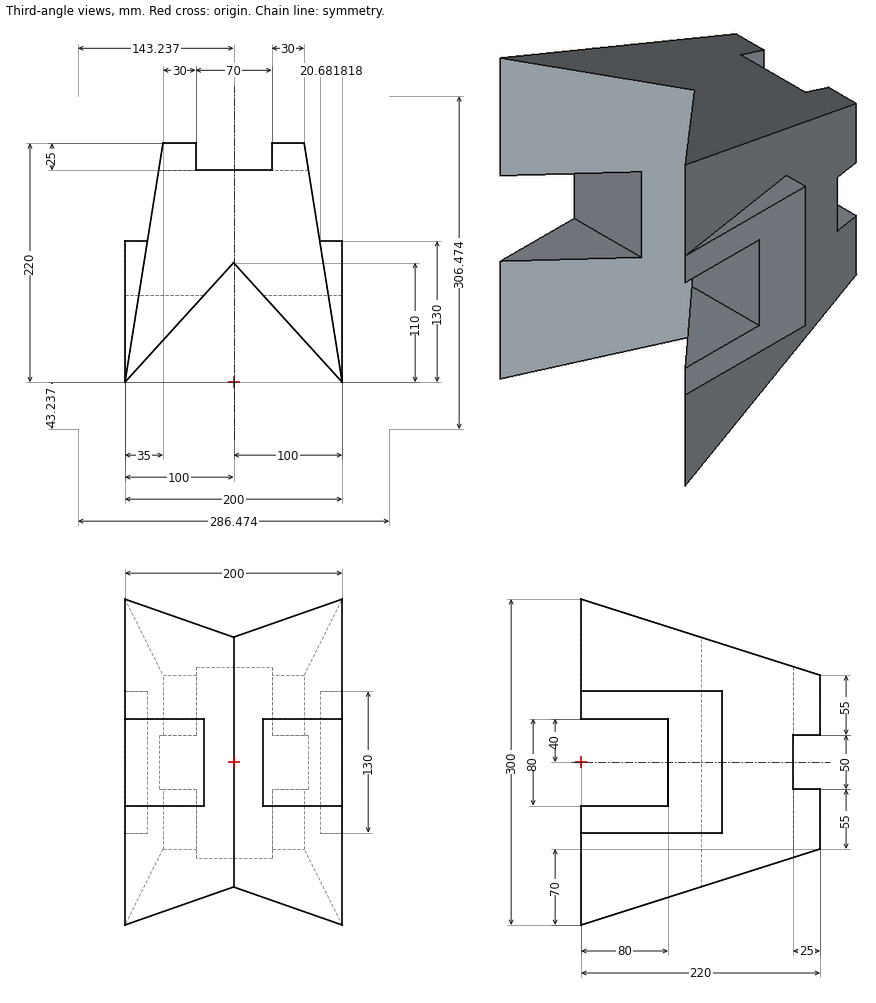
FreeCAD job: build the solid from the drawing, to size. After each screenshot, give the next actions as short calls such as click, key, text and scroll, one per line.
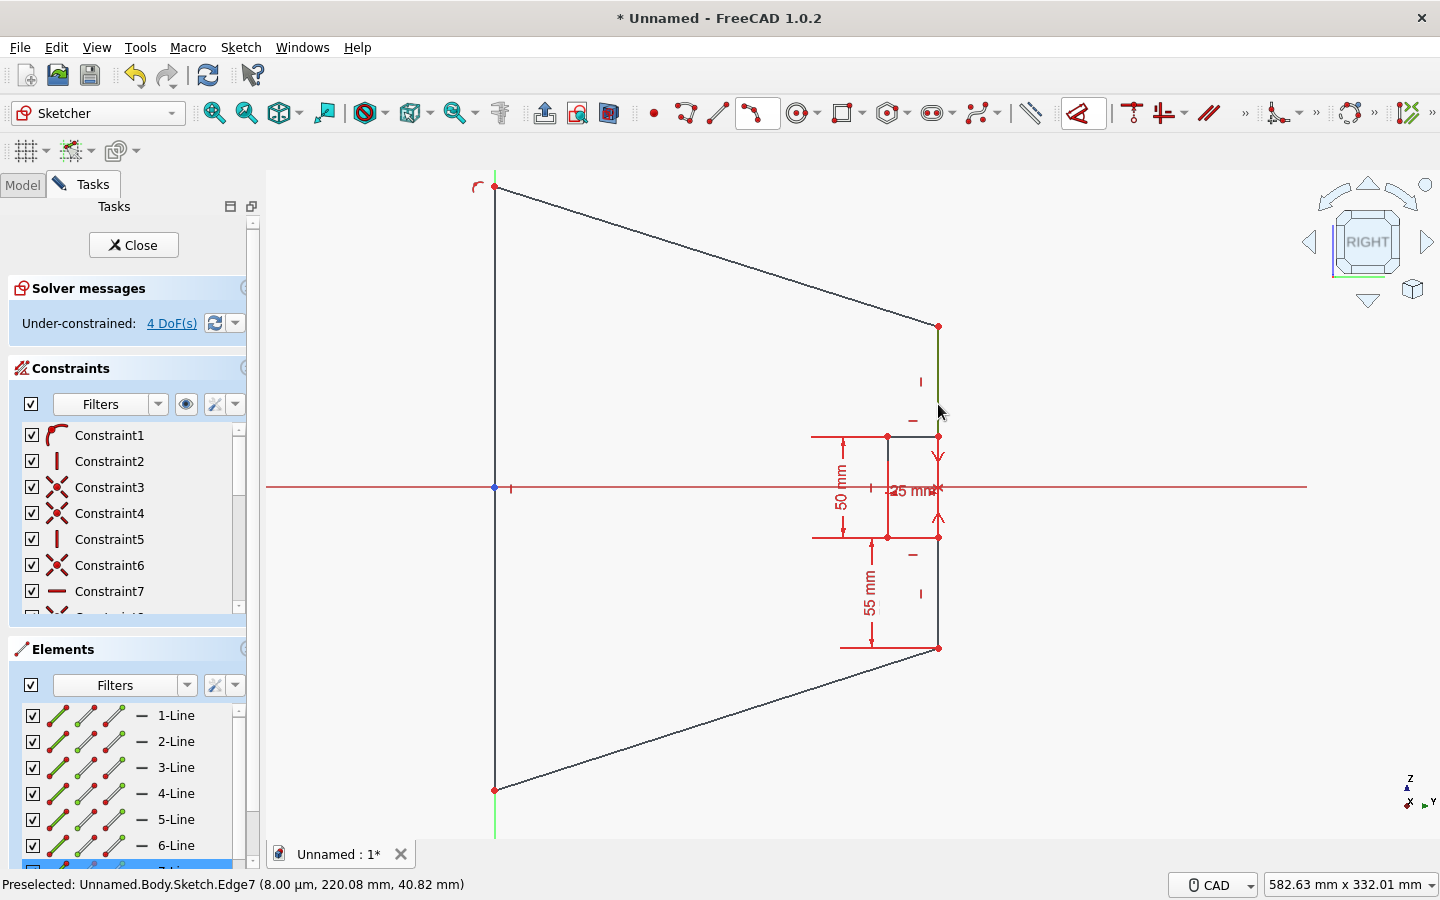
key(i)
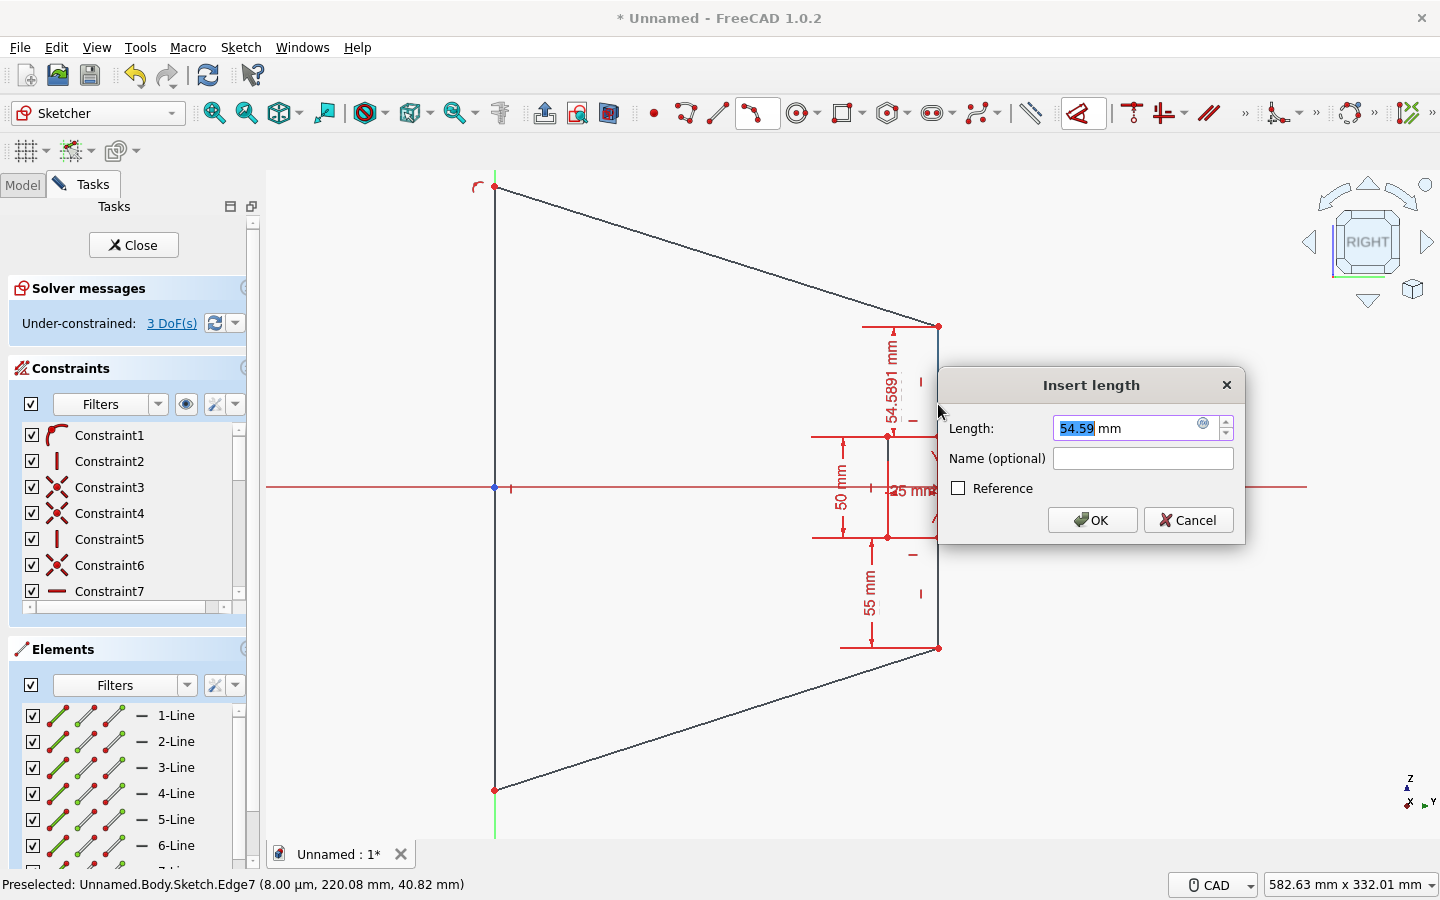
text(55)
key(Return)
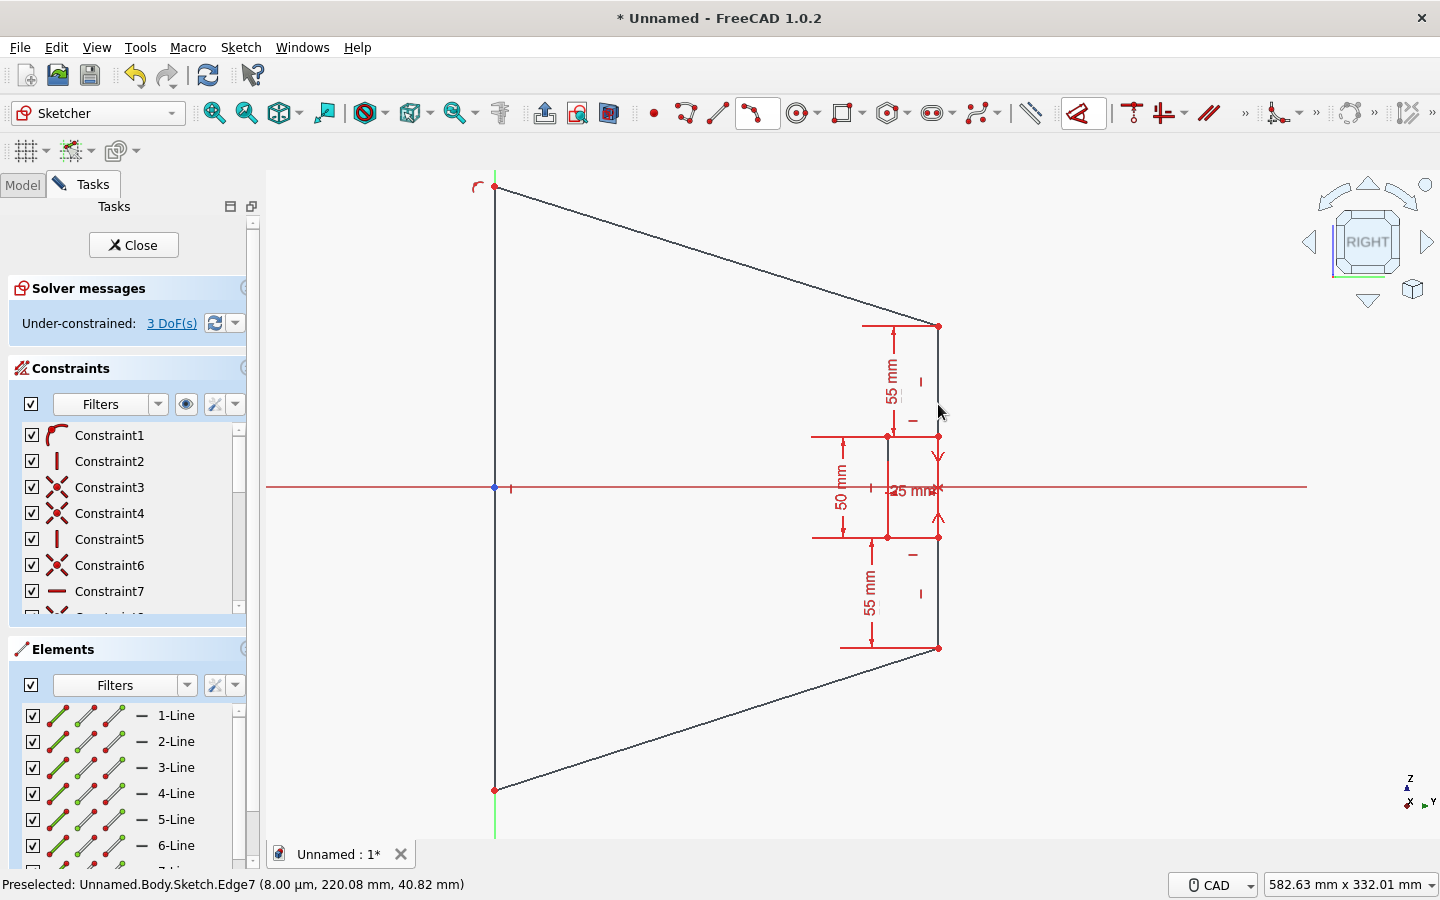
click(495, 368)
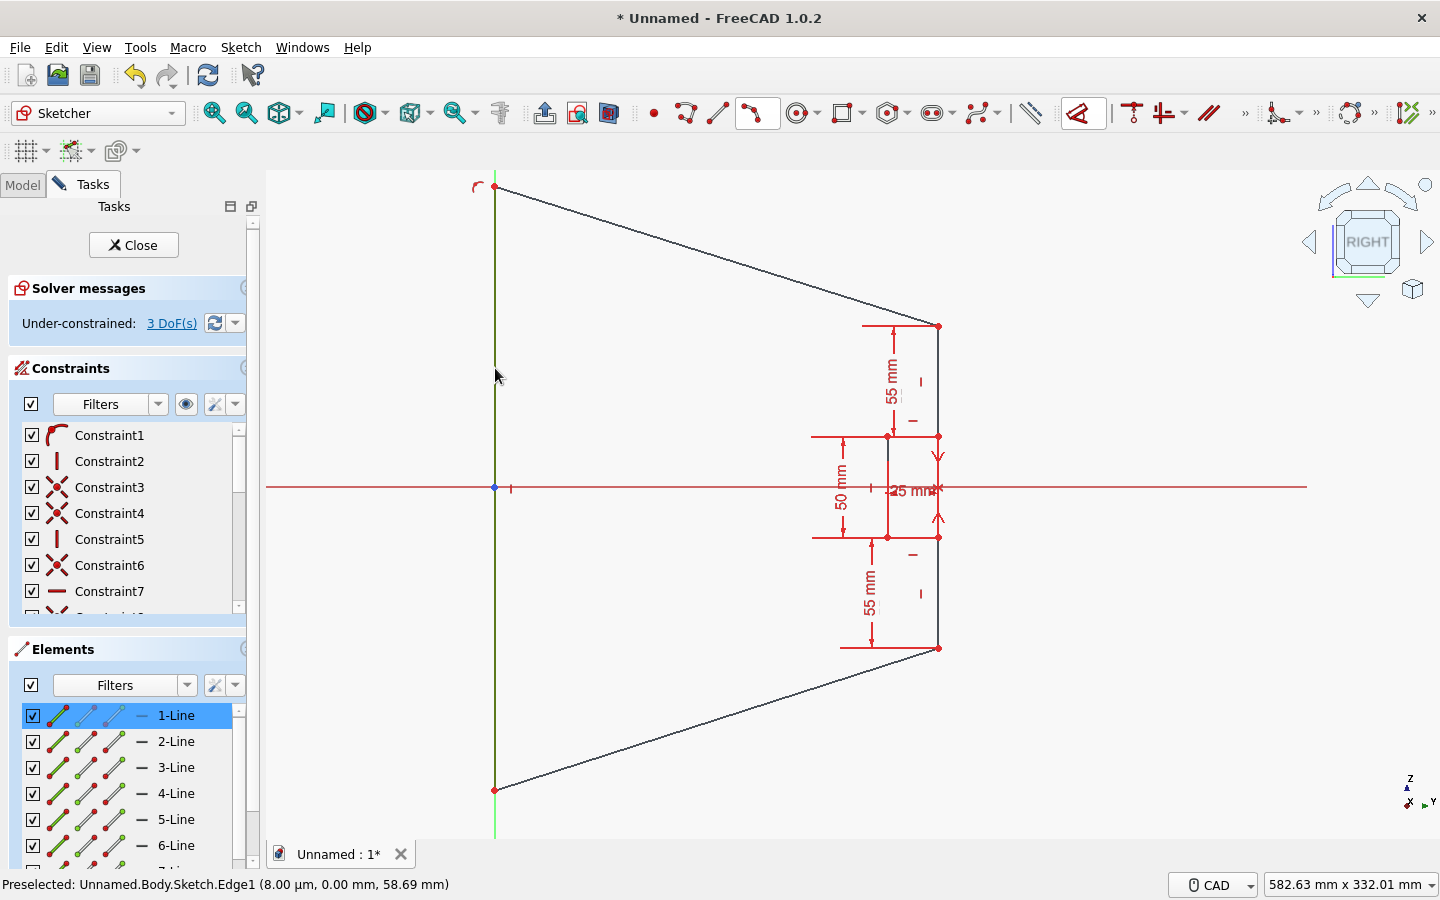
key(i)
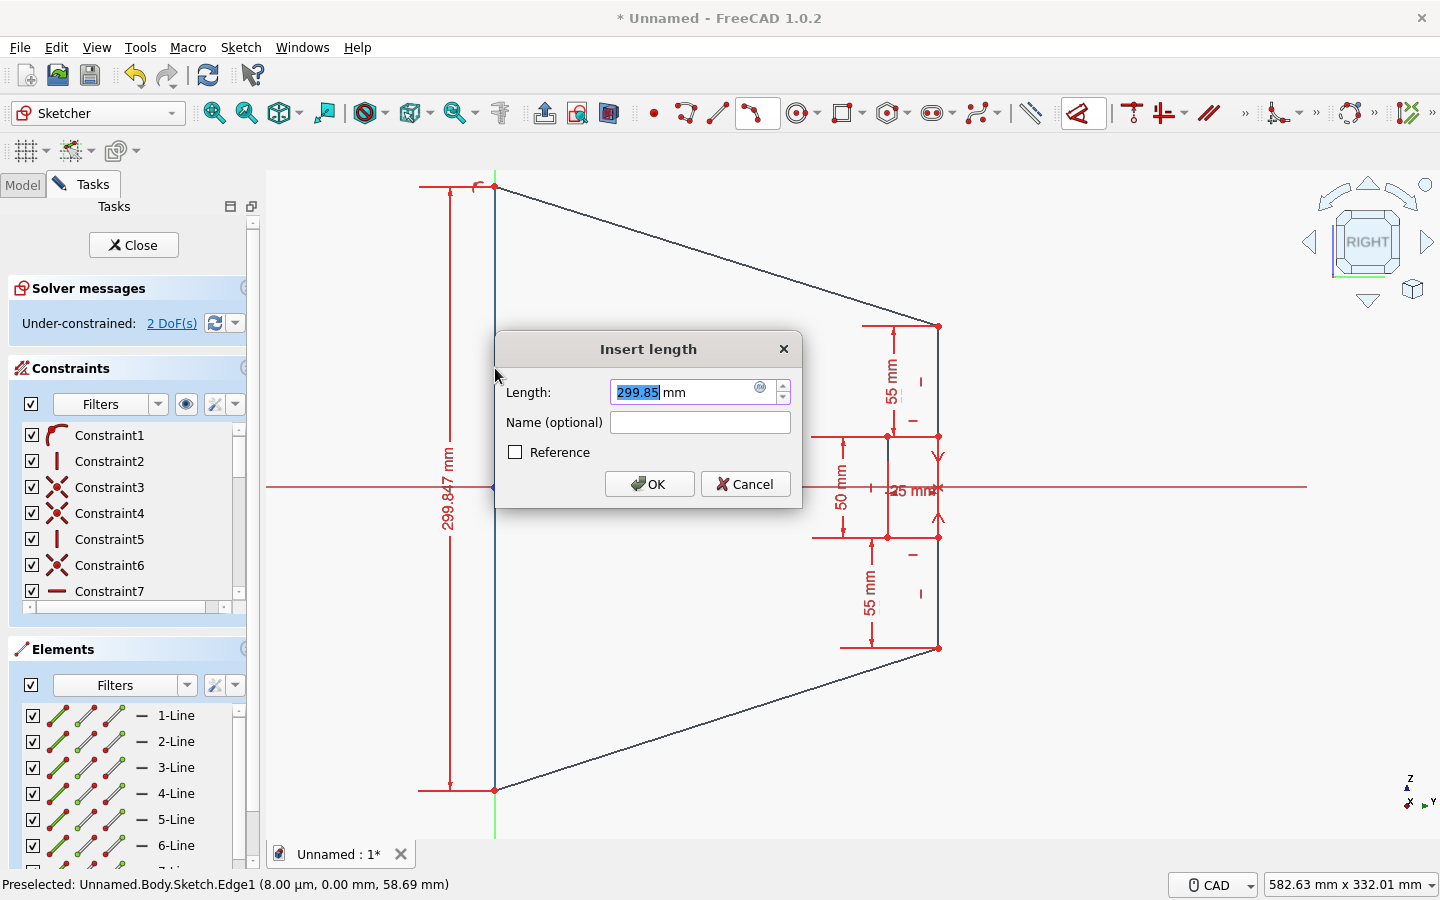
text(300)
key(Return)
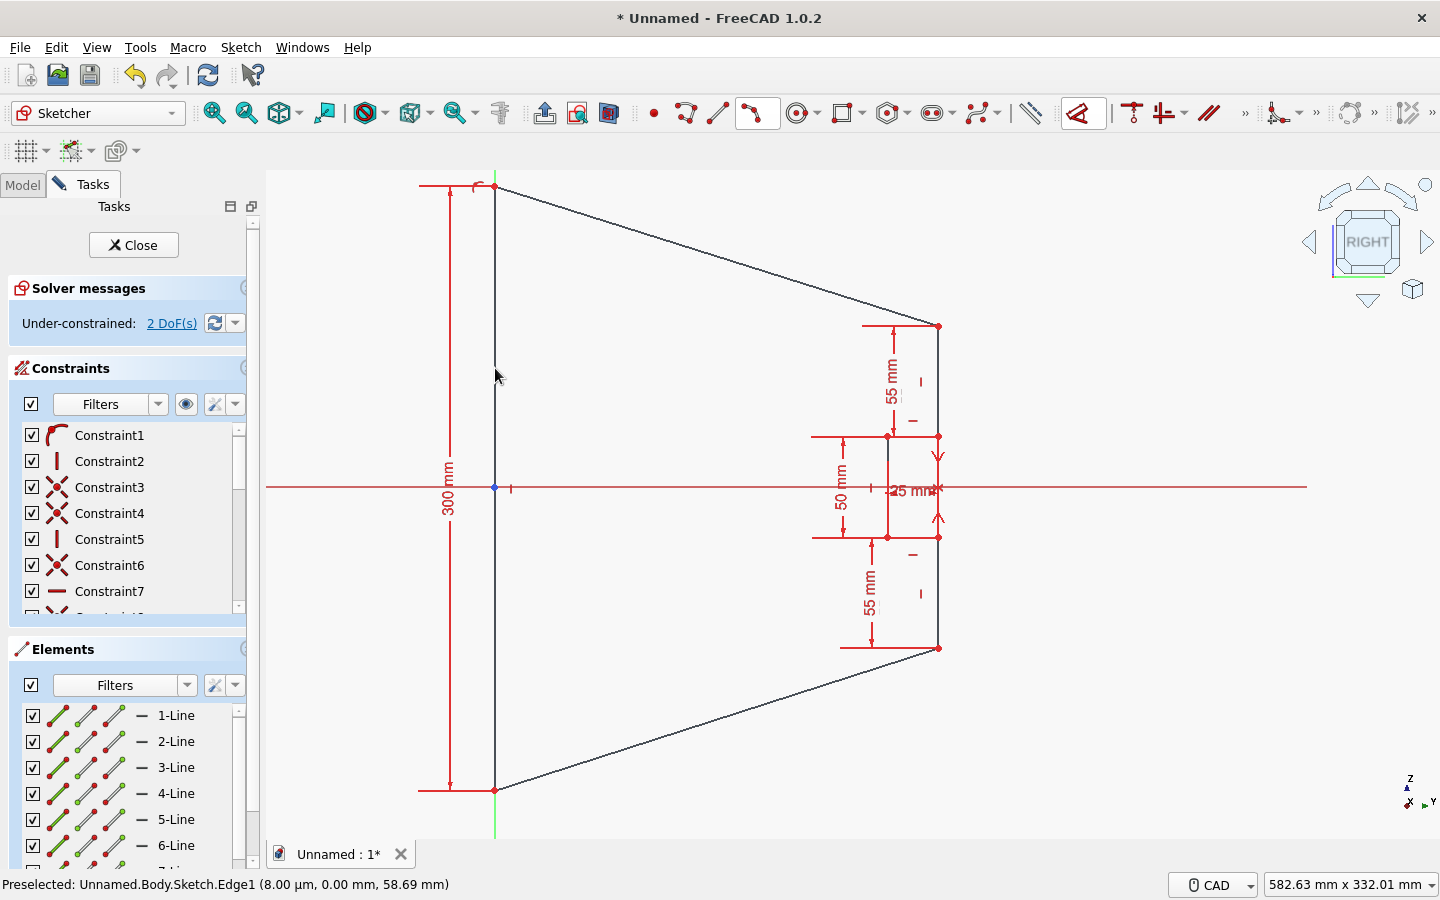
click(628, 748)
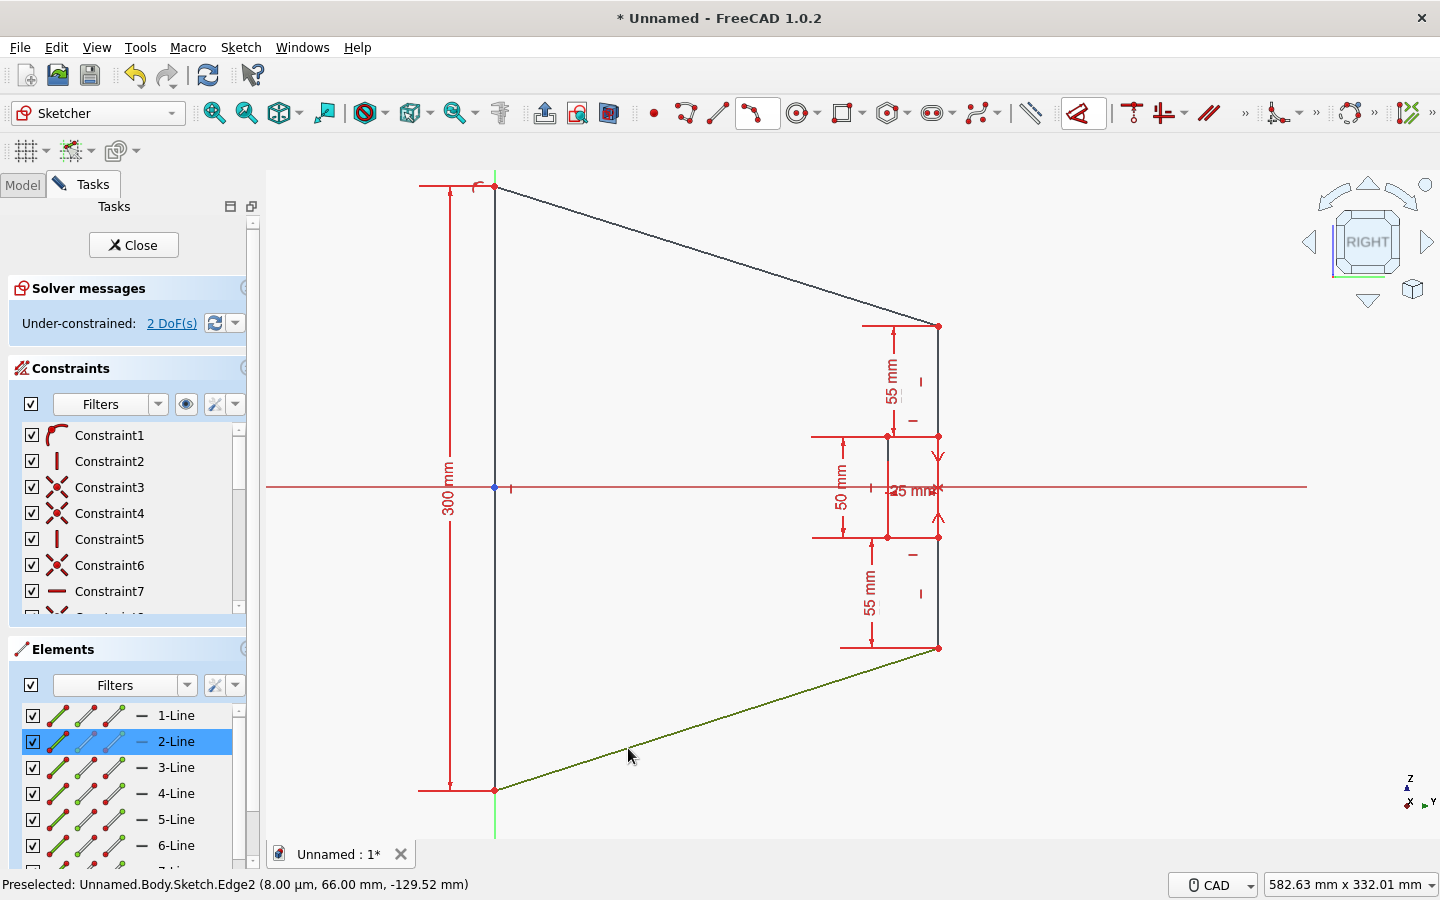
key(i)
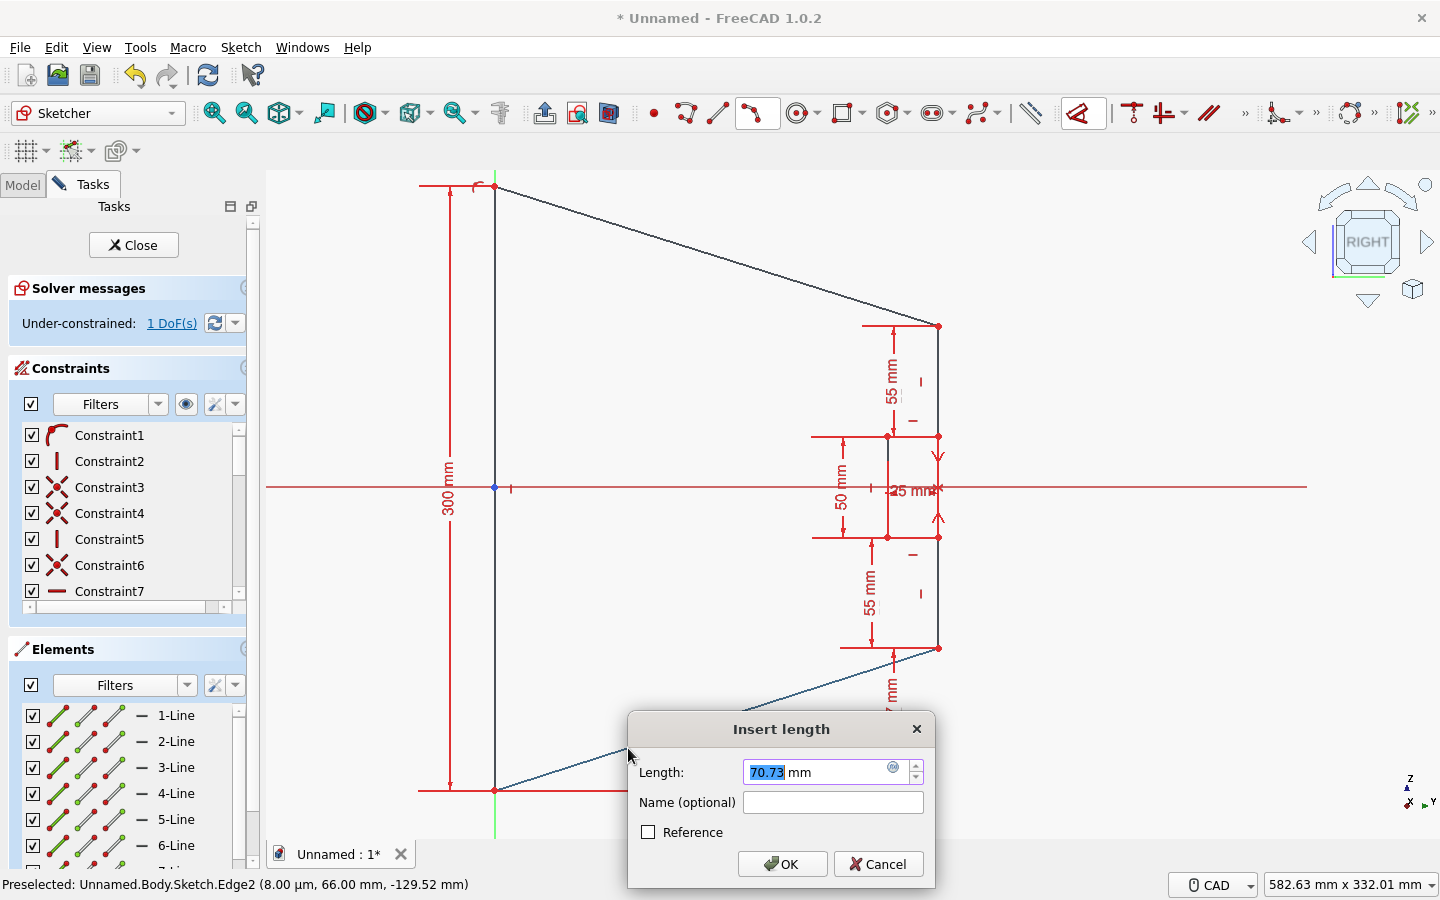
text(70)
key(Return)